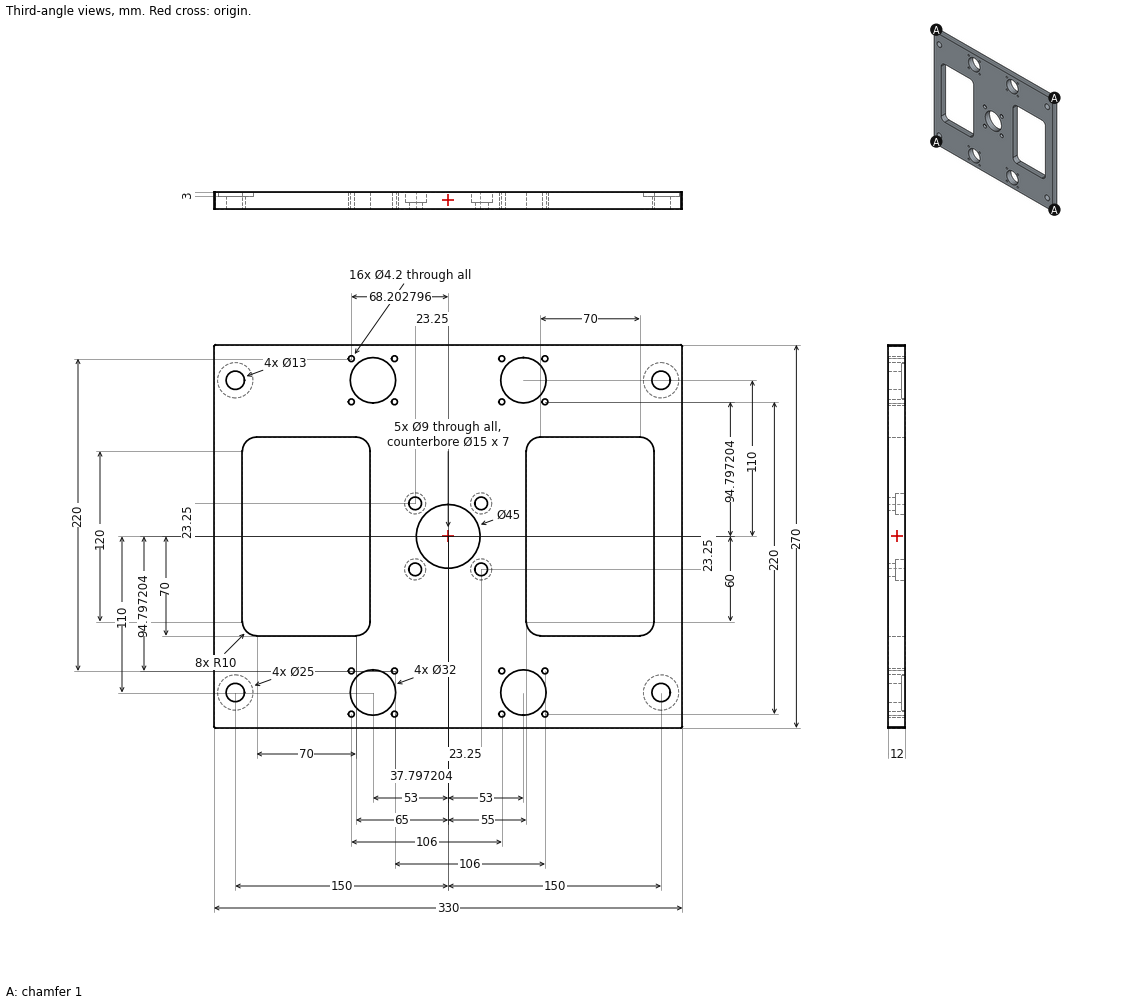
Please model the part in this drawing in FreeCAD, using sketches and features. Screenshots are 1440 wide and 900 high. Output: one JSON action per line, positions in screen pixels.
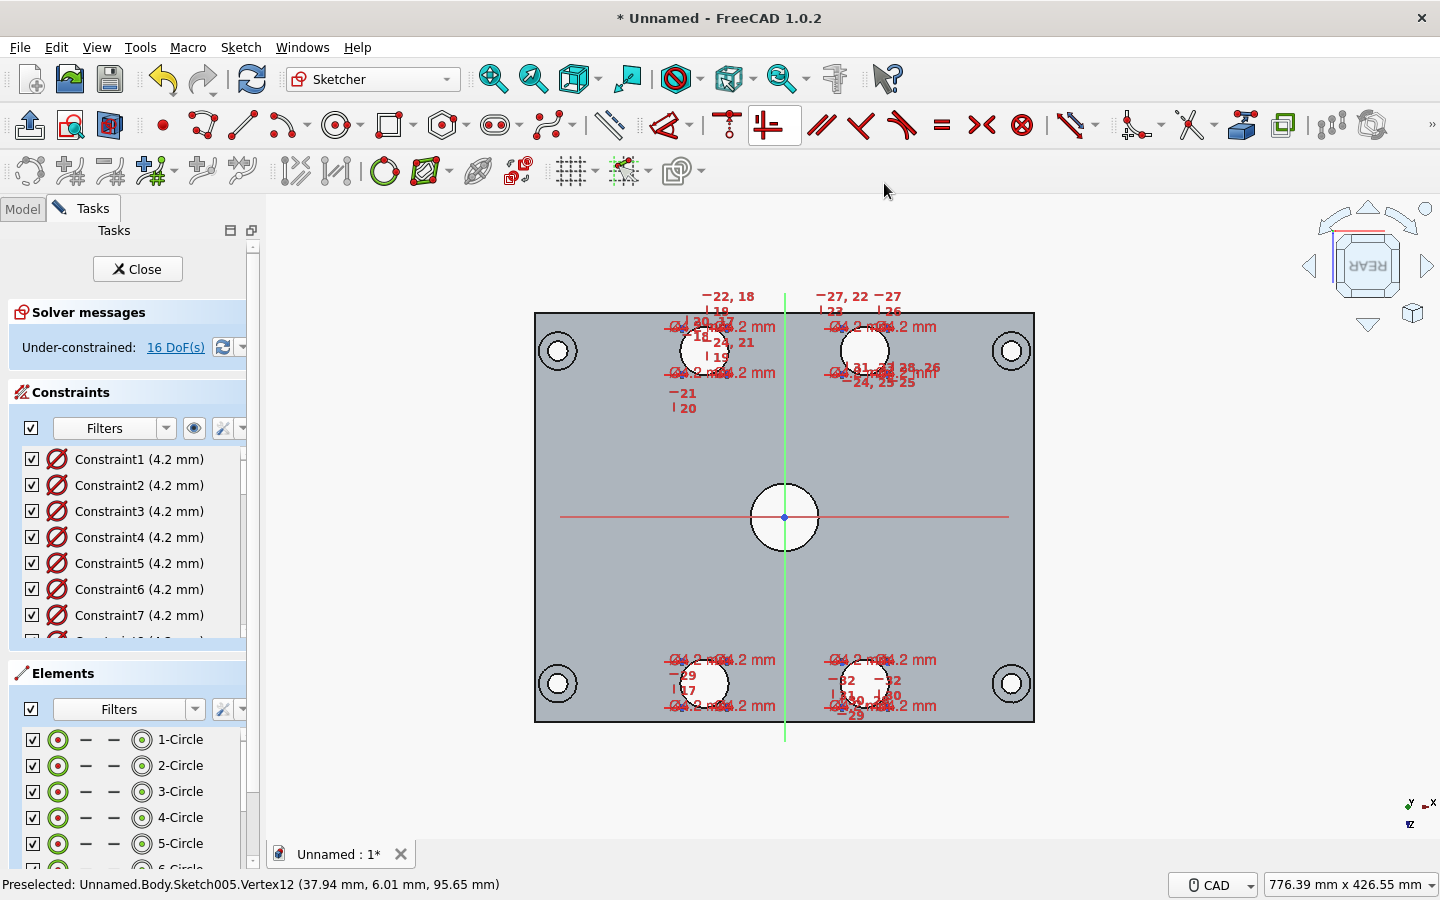
{"action": "left_click", "coordinate": [842, 662]}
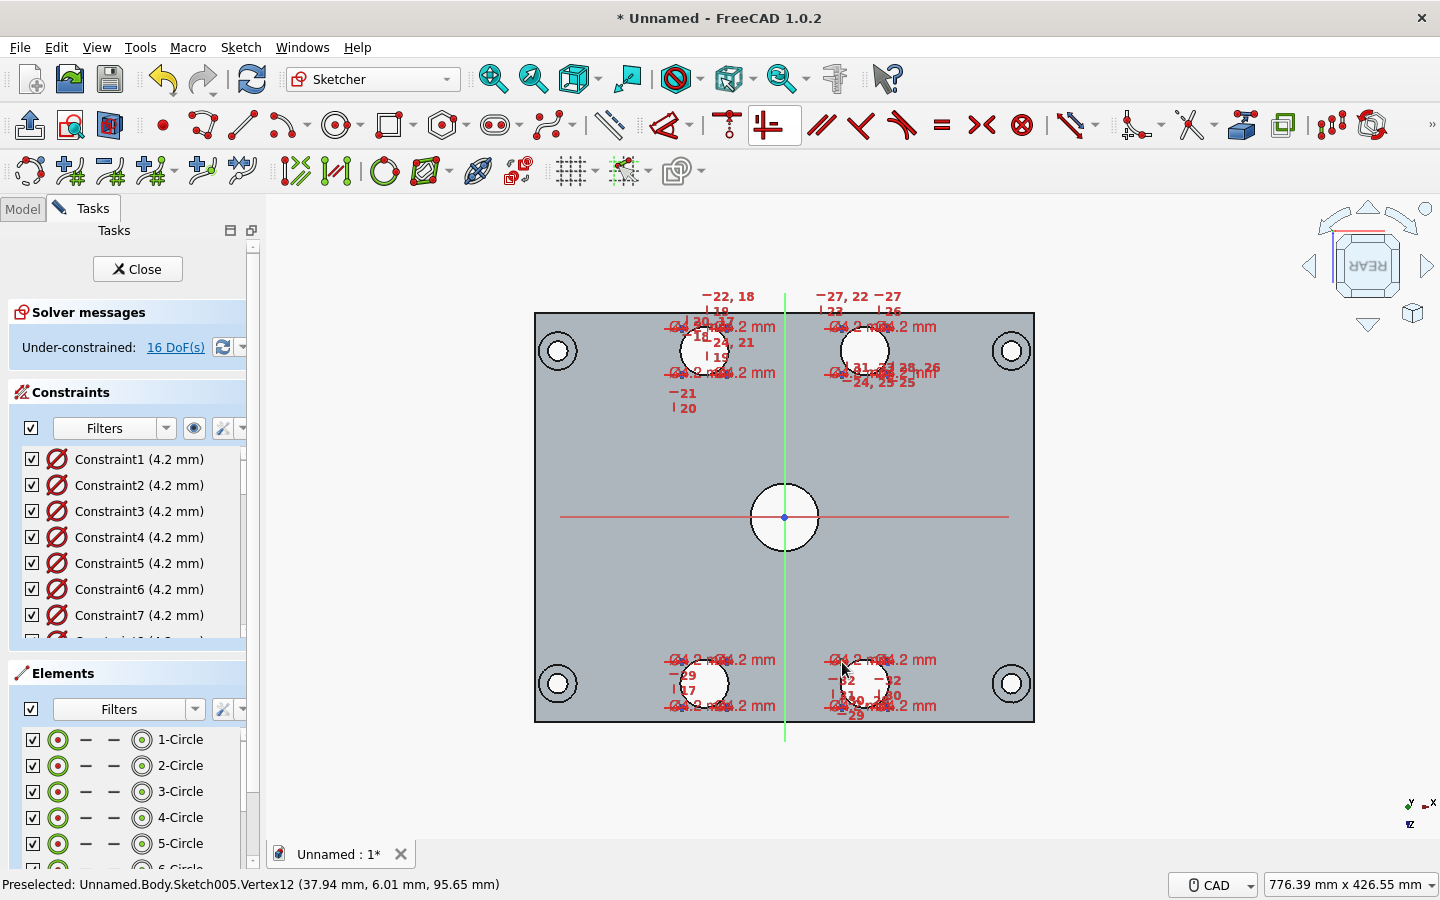
{"action": "left_click", "coordinate": [842, 708]}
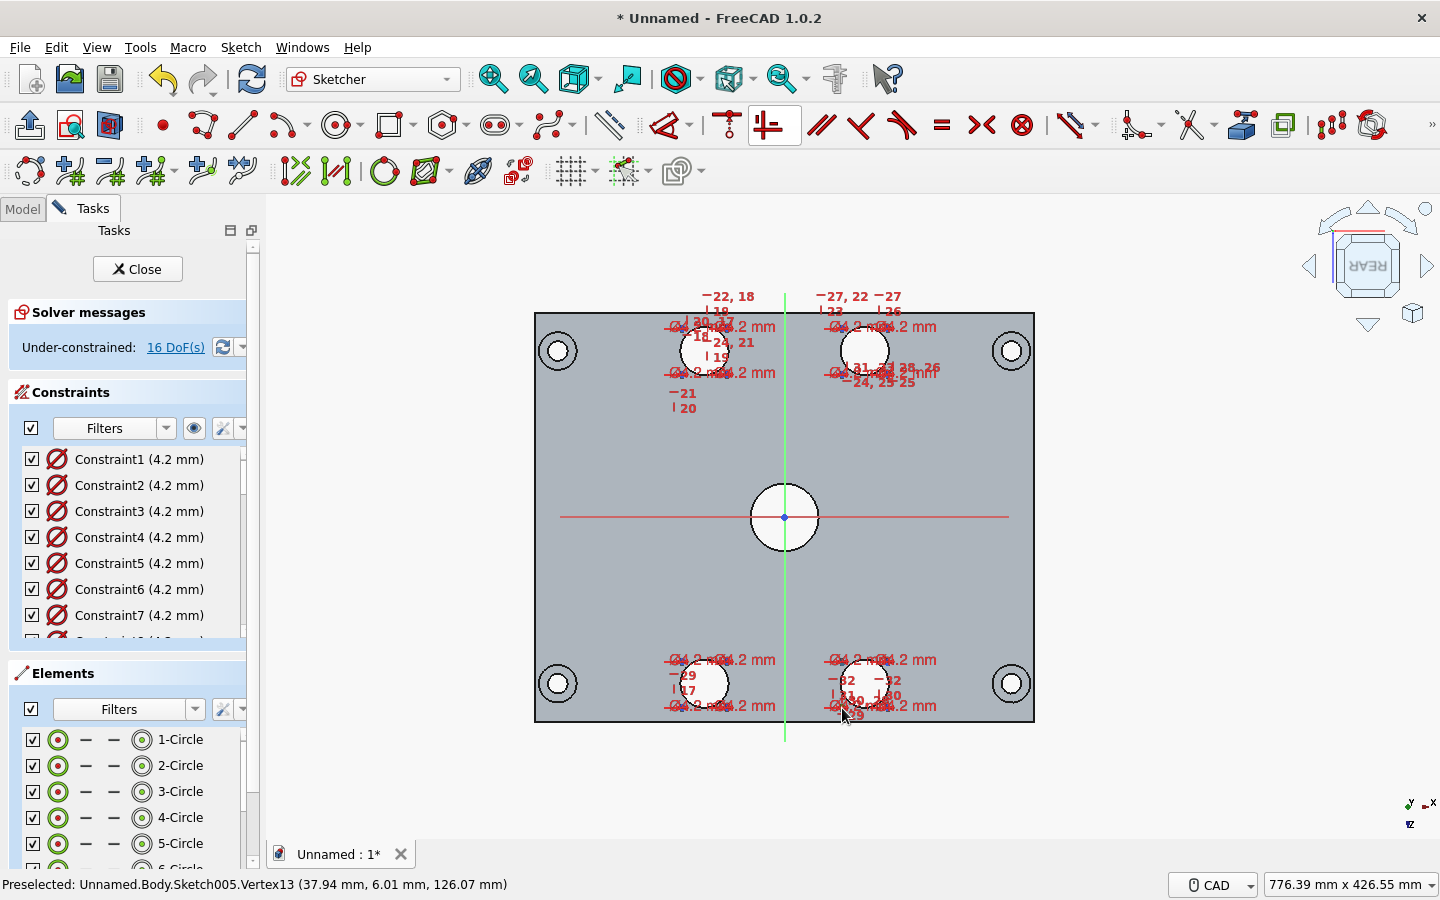
{"action": "key", "text": "v"}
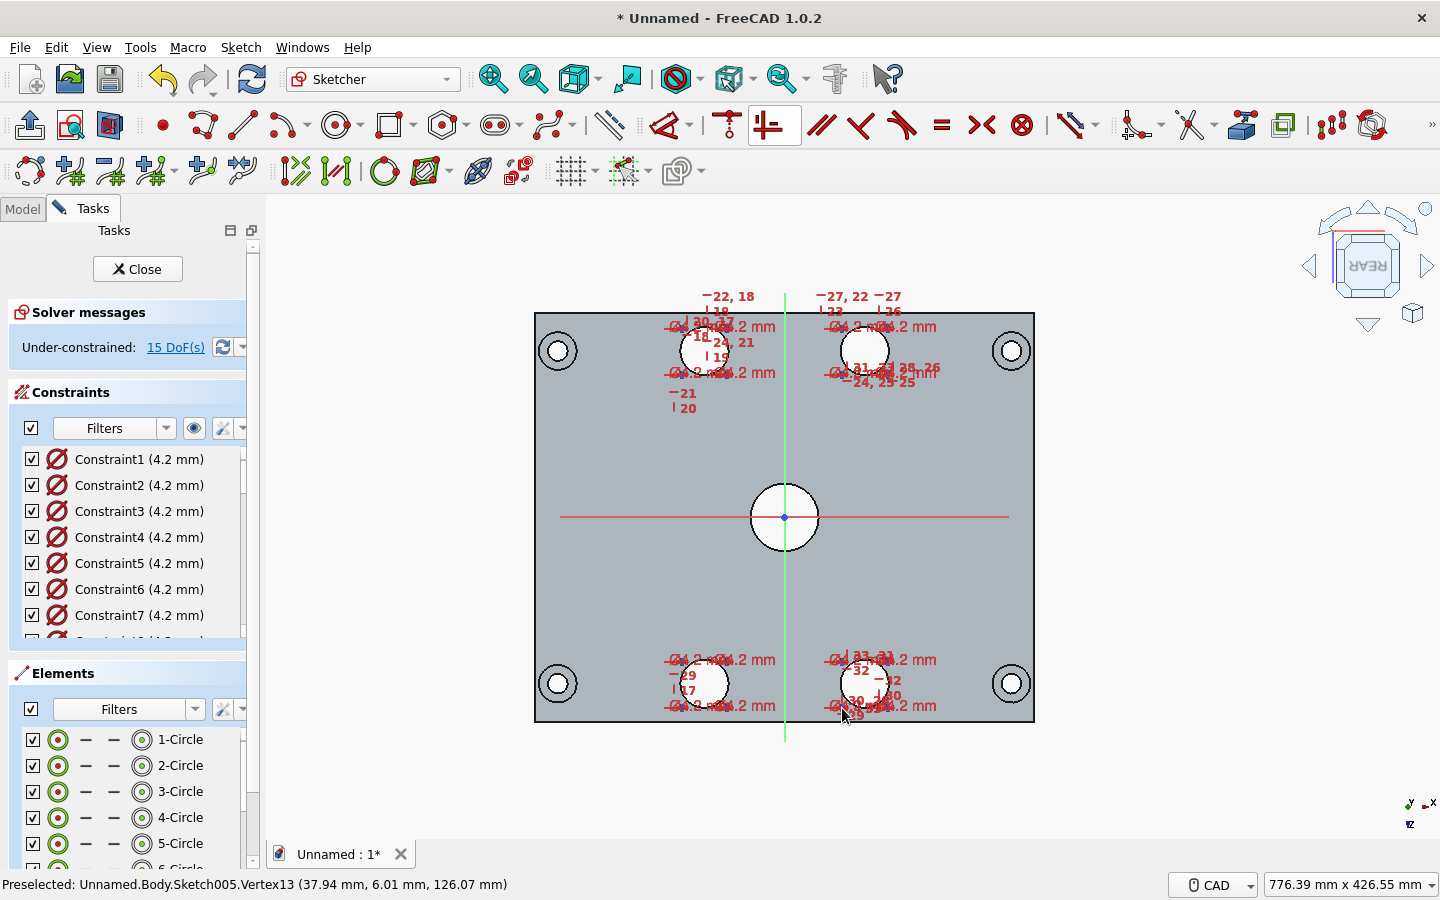
{"action": "left_click", "coordinate": [888, 708]}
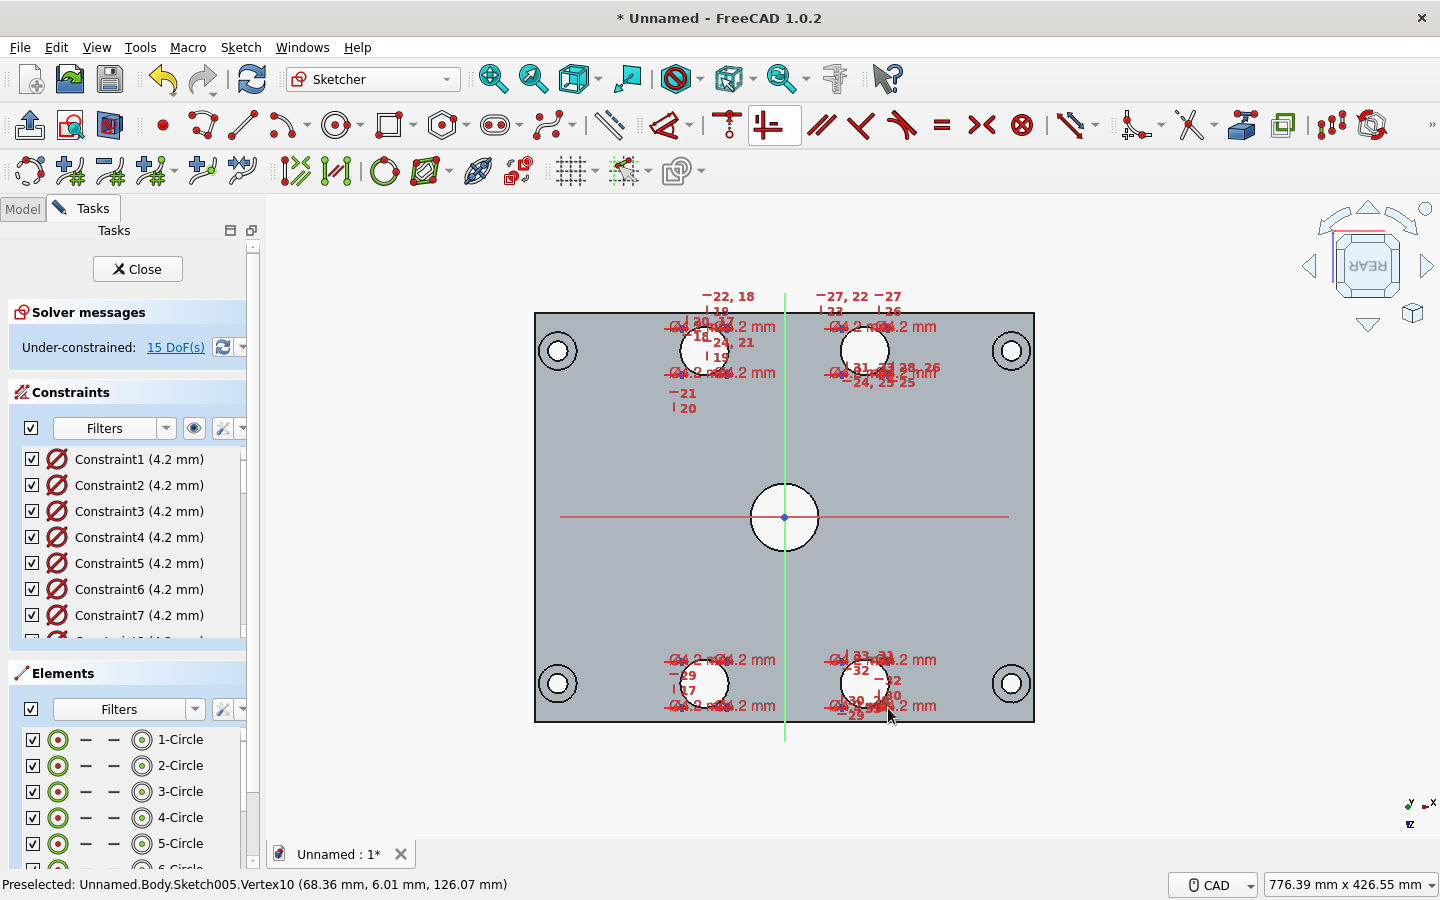
{"action": "left_click", "coordinate": [842, 708]}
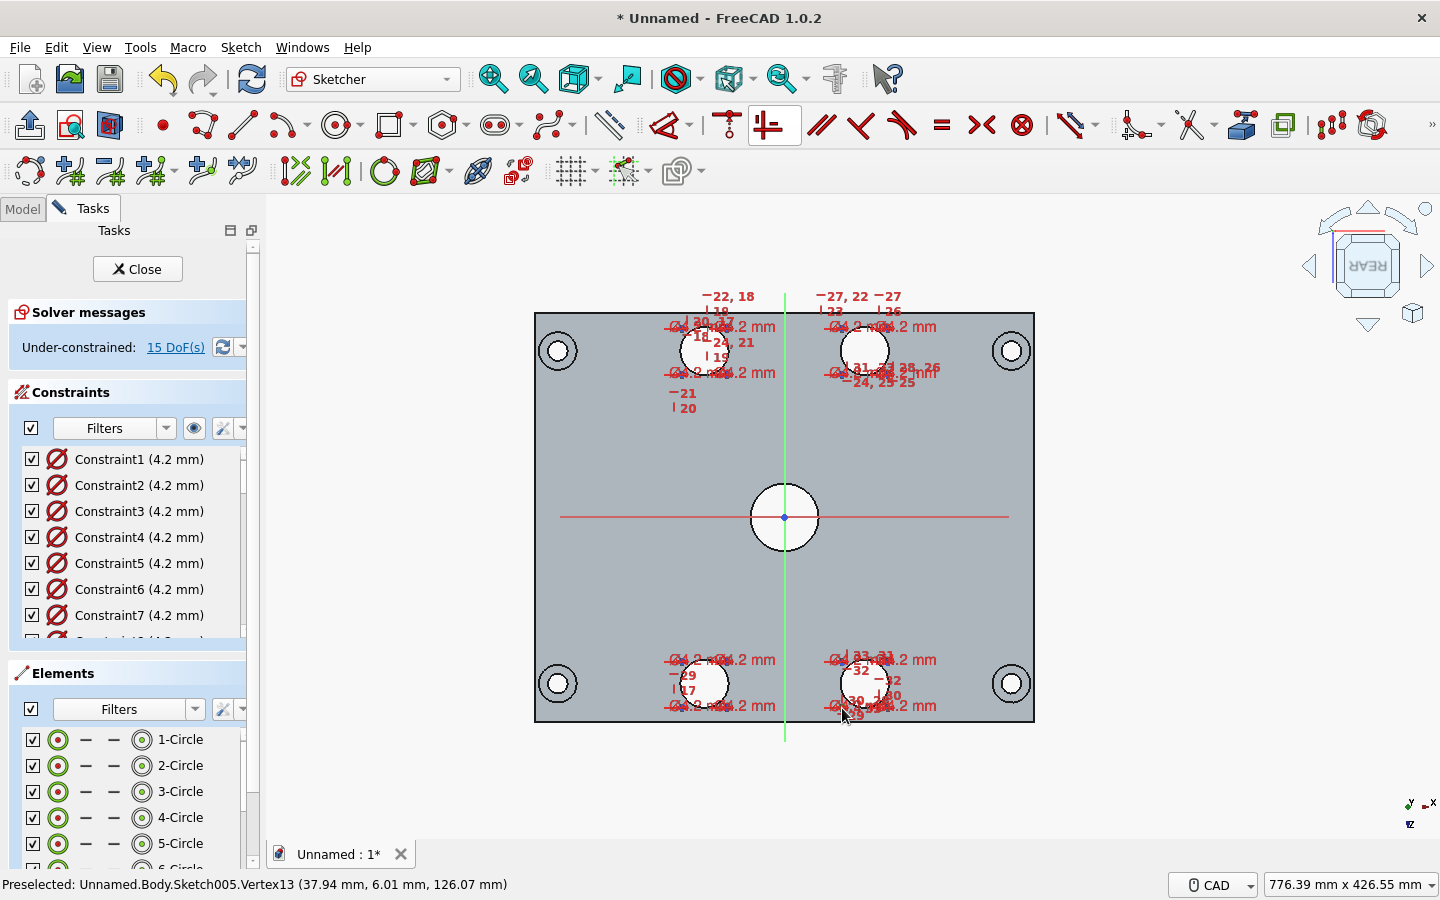
{"action": "left_click", "coordinate": [796, 126]}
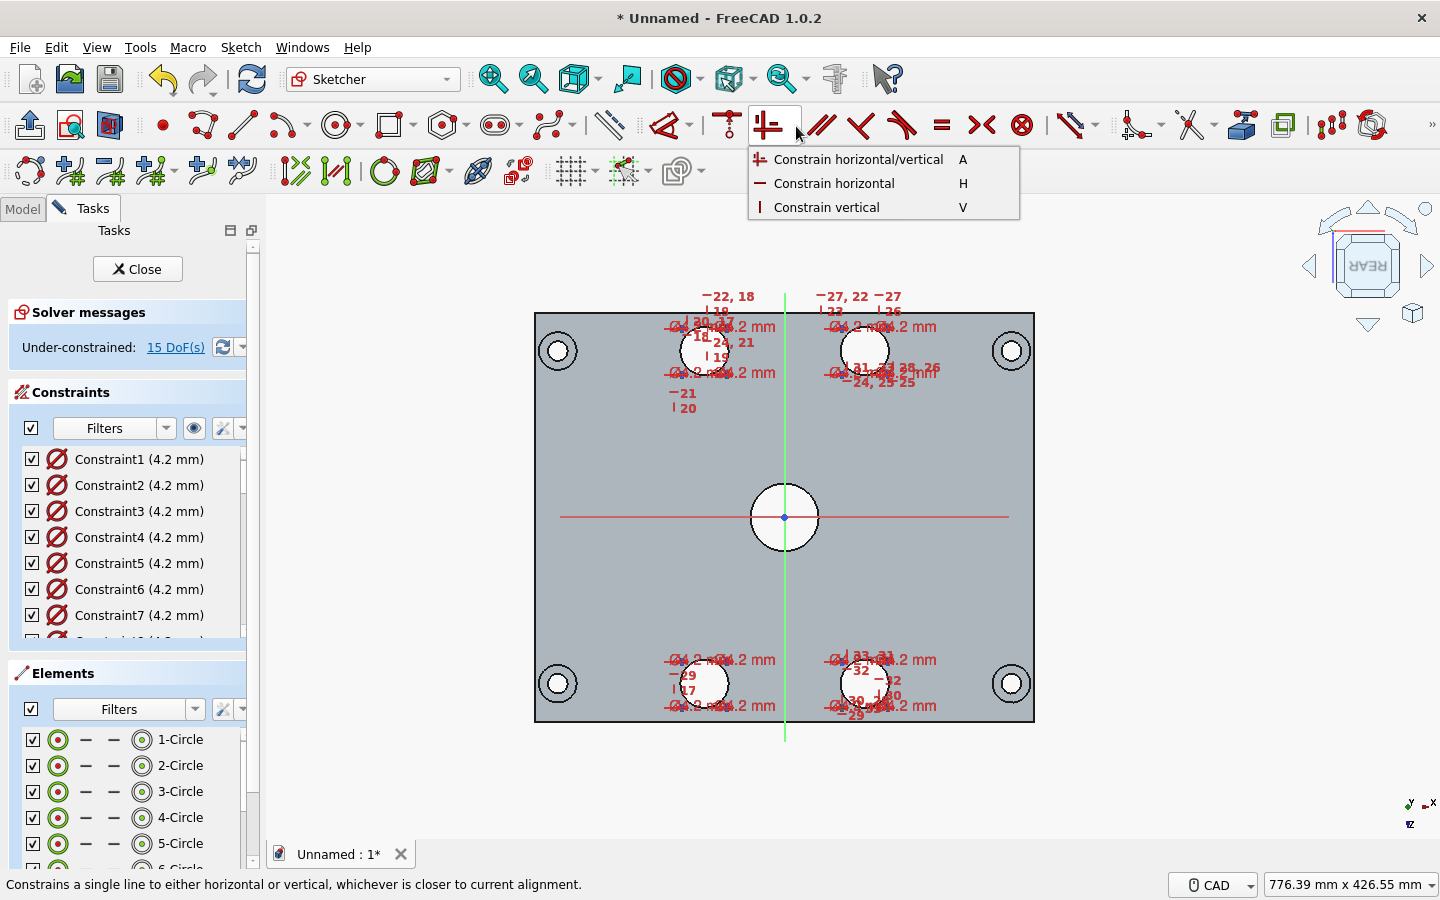
{"action": "left_click", "coordinate": [884, 183]}